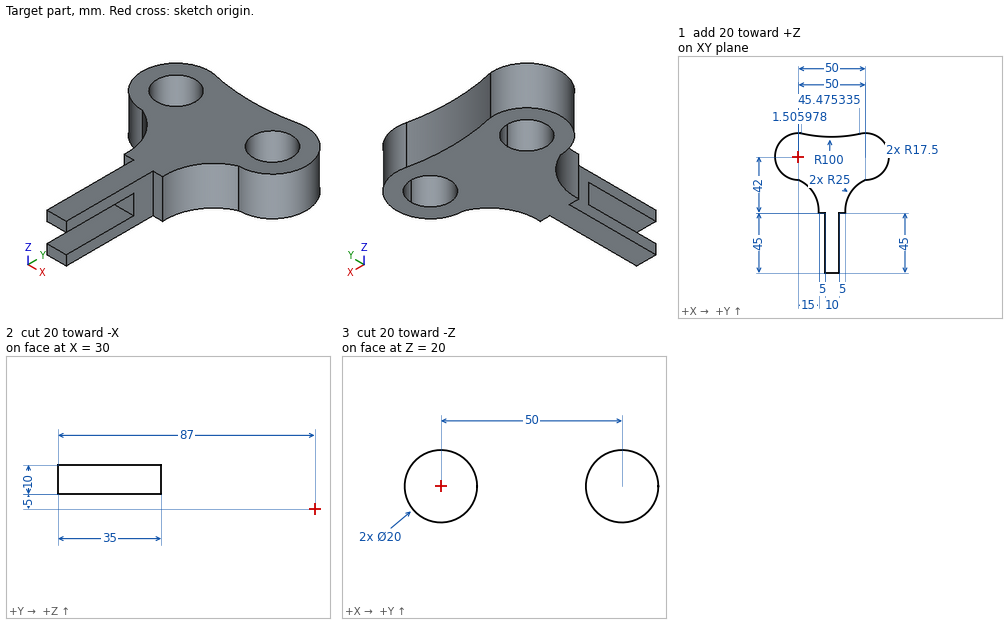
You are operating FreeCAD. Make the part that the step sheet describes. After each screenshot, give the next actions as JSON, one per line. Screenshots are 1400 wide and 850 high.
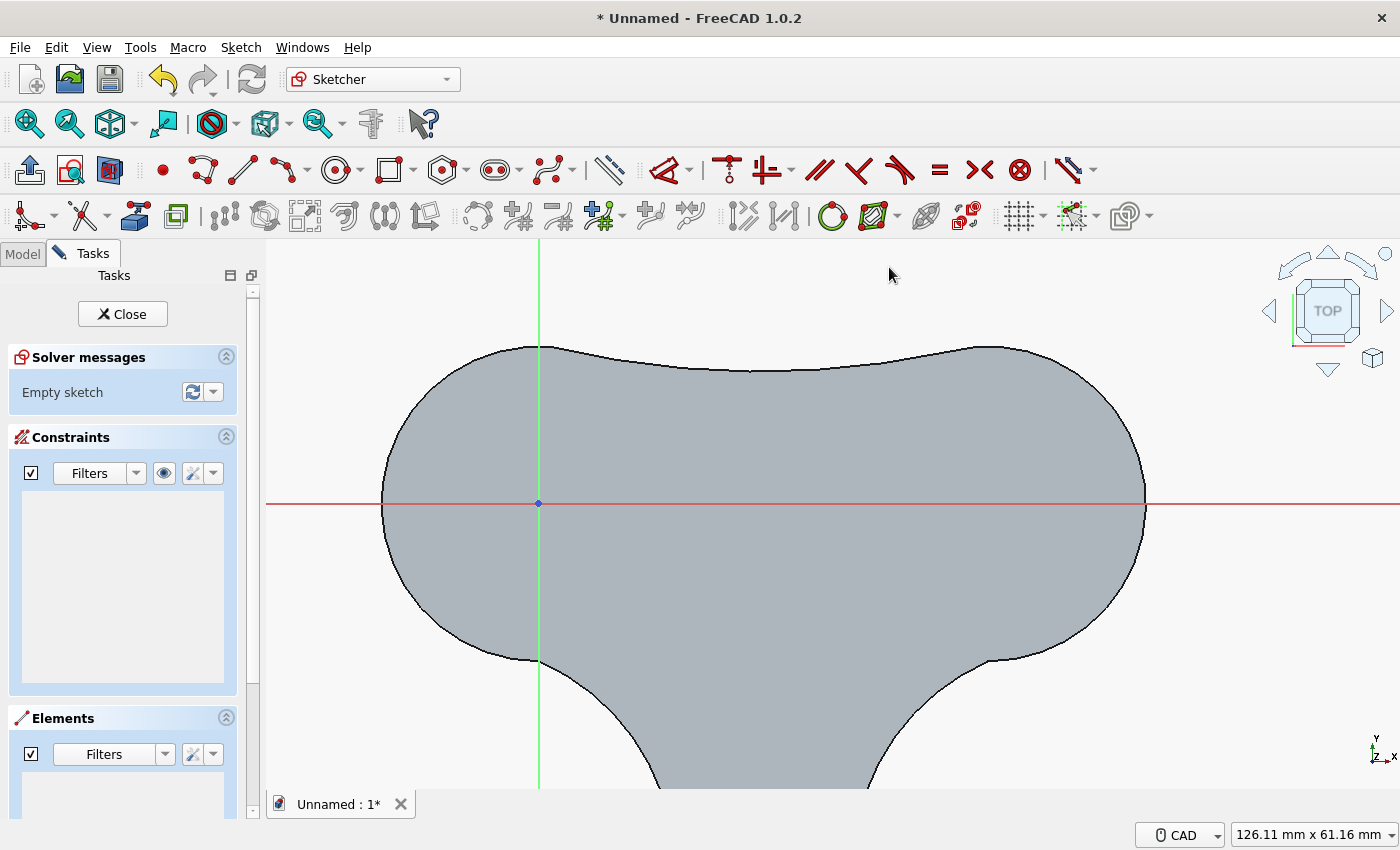
{"action": "left_click", "coordinate": [336, 170]}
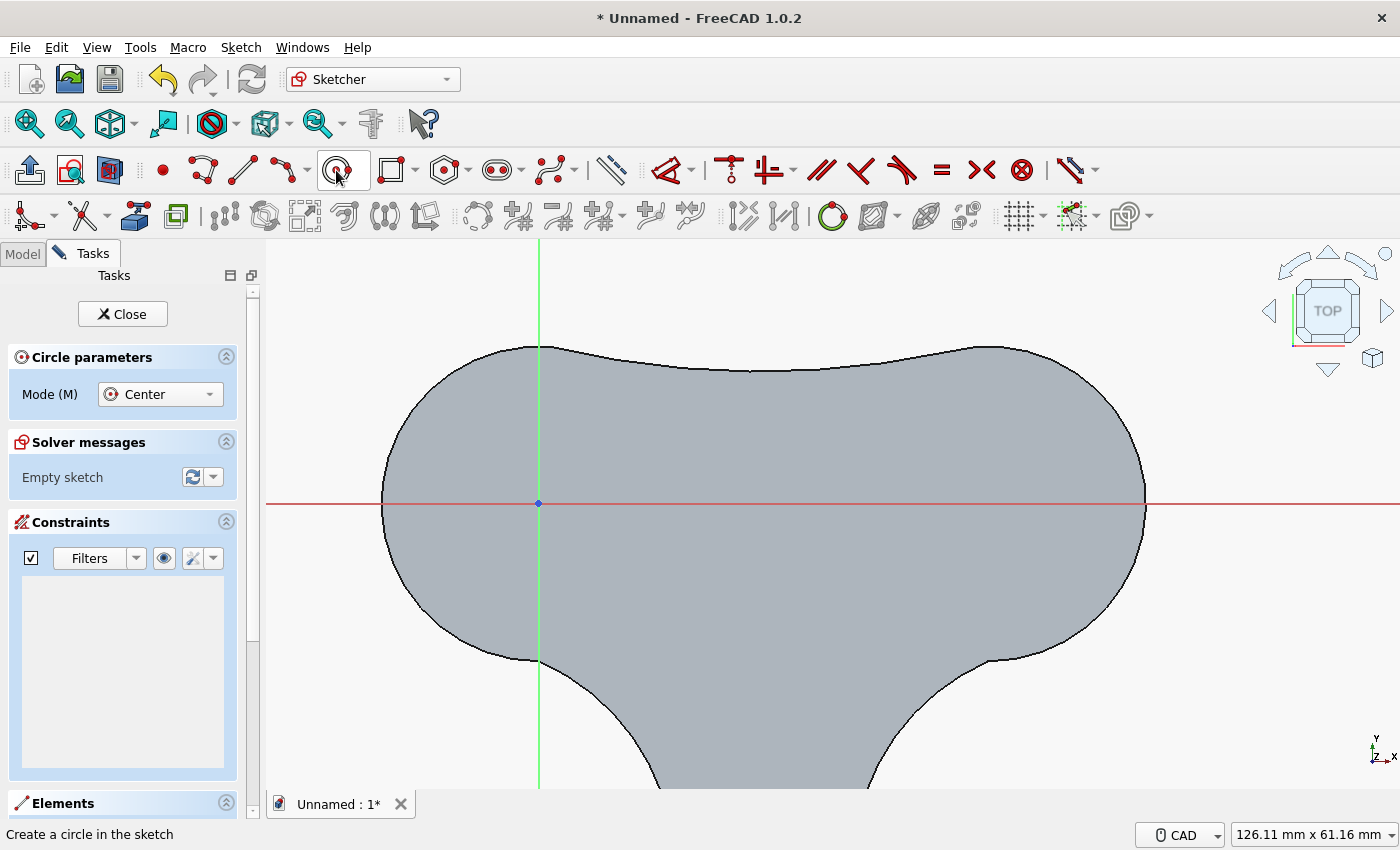
{"action": "left_click", "coordinate": [539, 504]}
{"action": "left_click", "coordinate": [602, 440]}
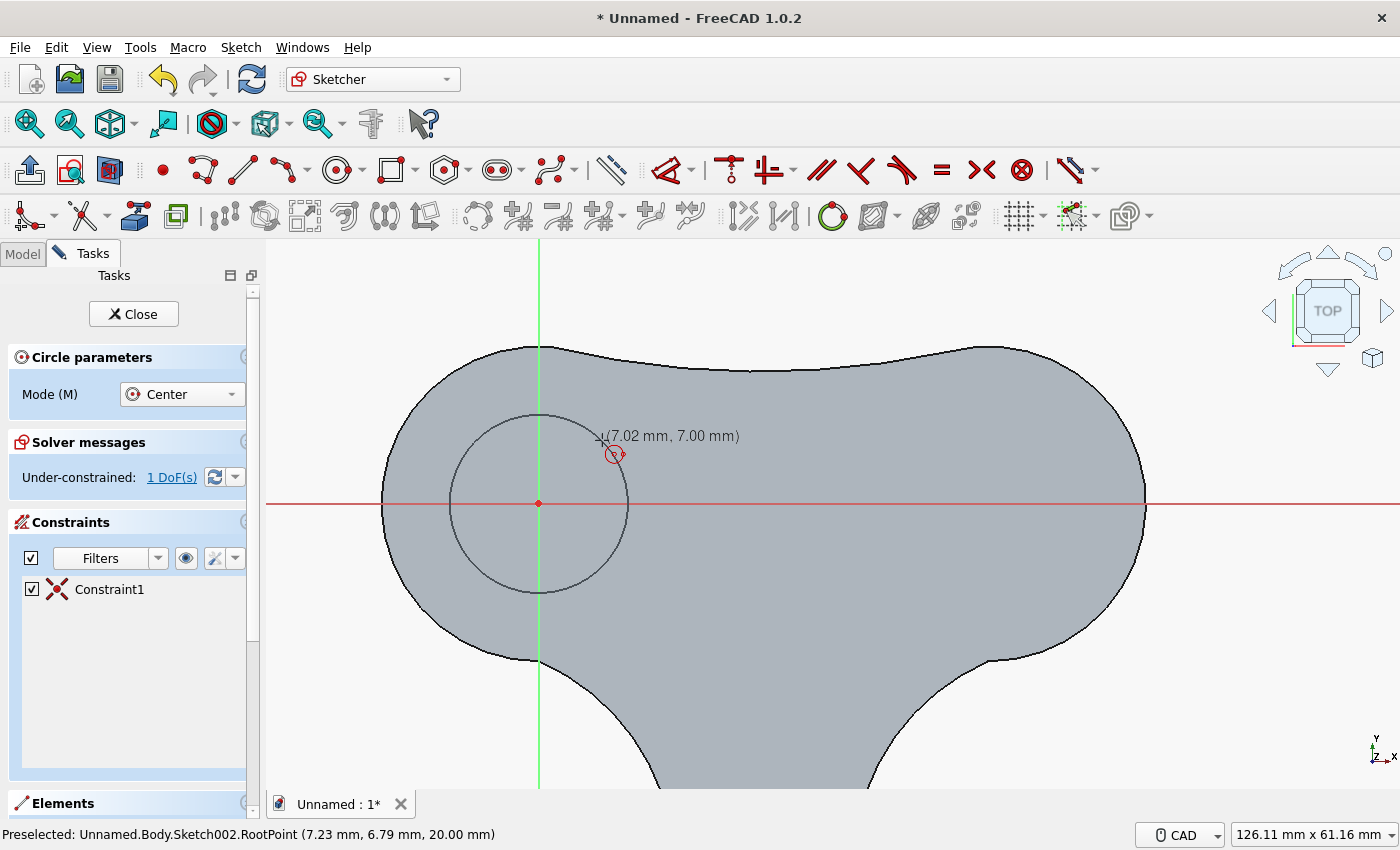
{"action": "left_click", "coordinate": [988, 504]}
{"action": "left_click", "coordinate": [1052, 440]}
{"action": "key", "text": "Escape"}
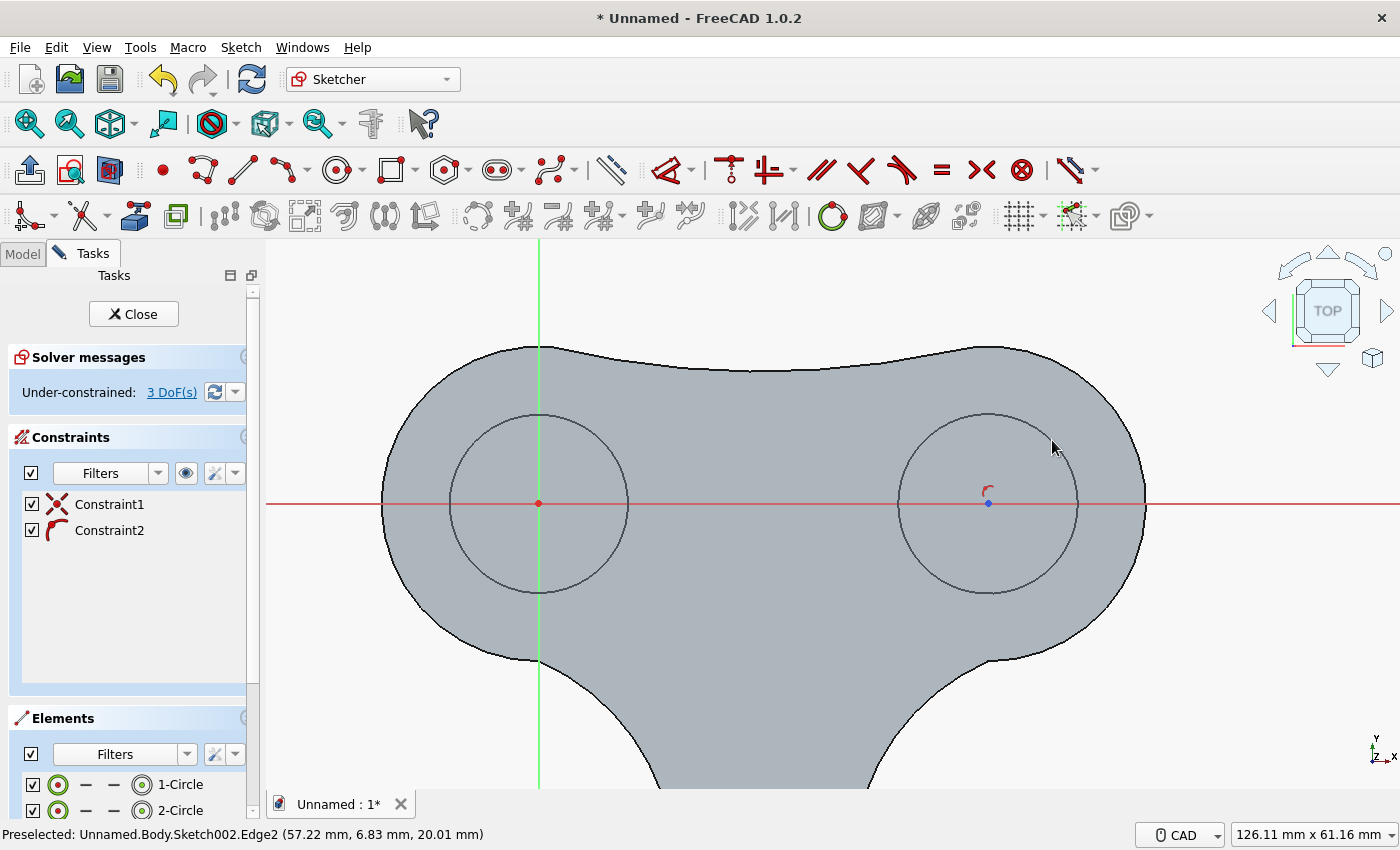
{"action": "left_click", "coordinate": [602, 441]}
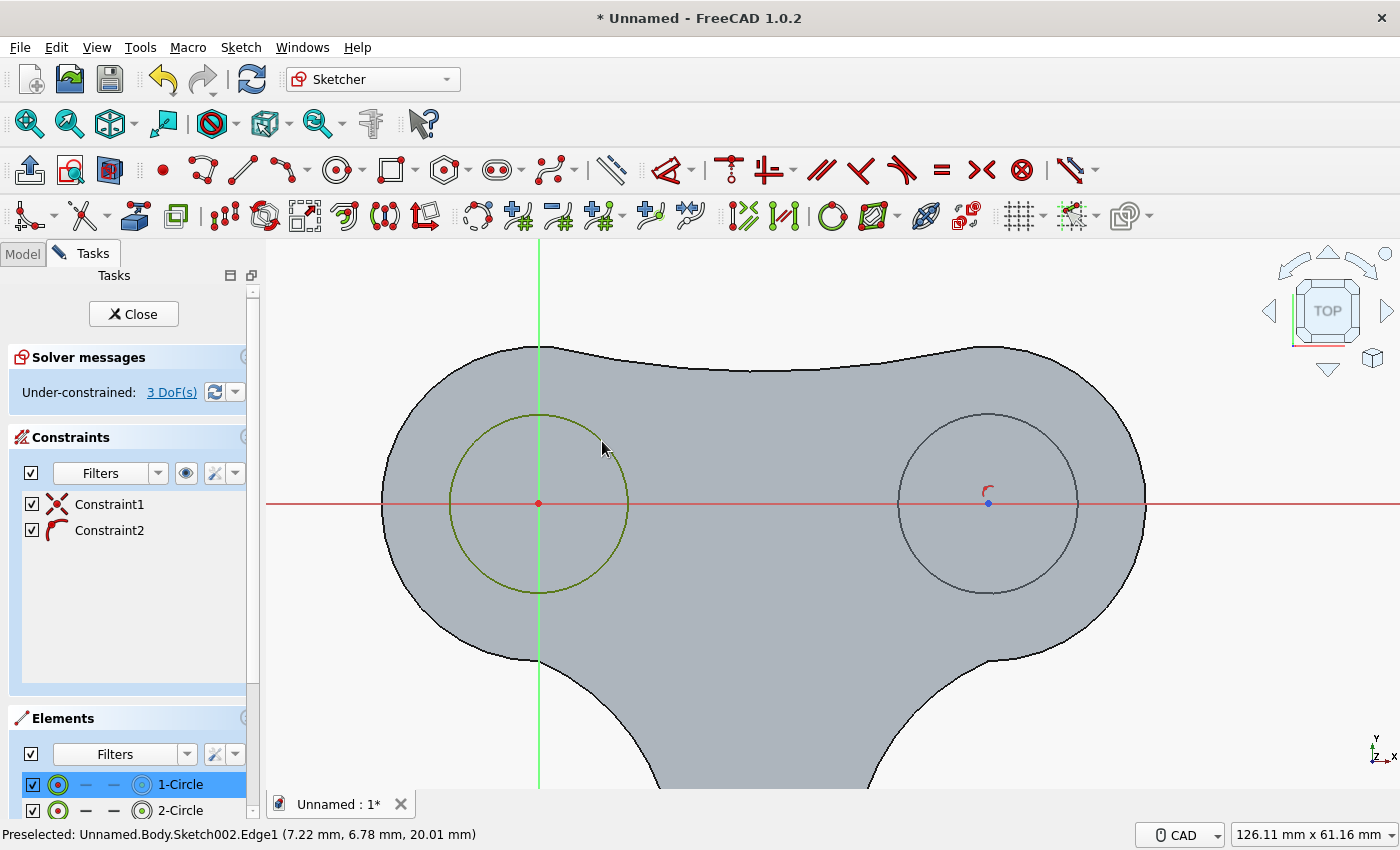
{"action": "left_click", "coordinate": [1051, 440]}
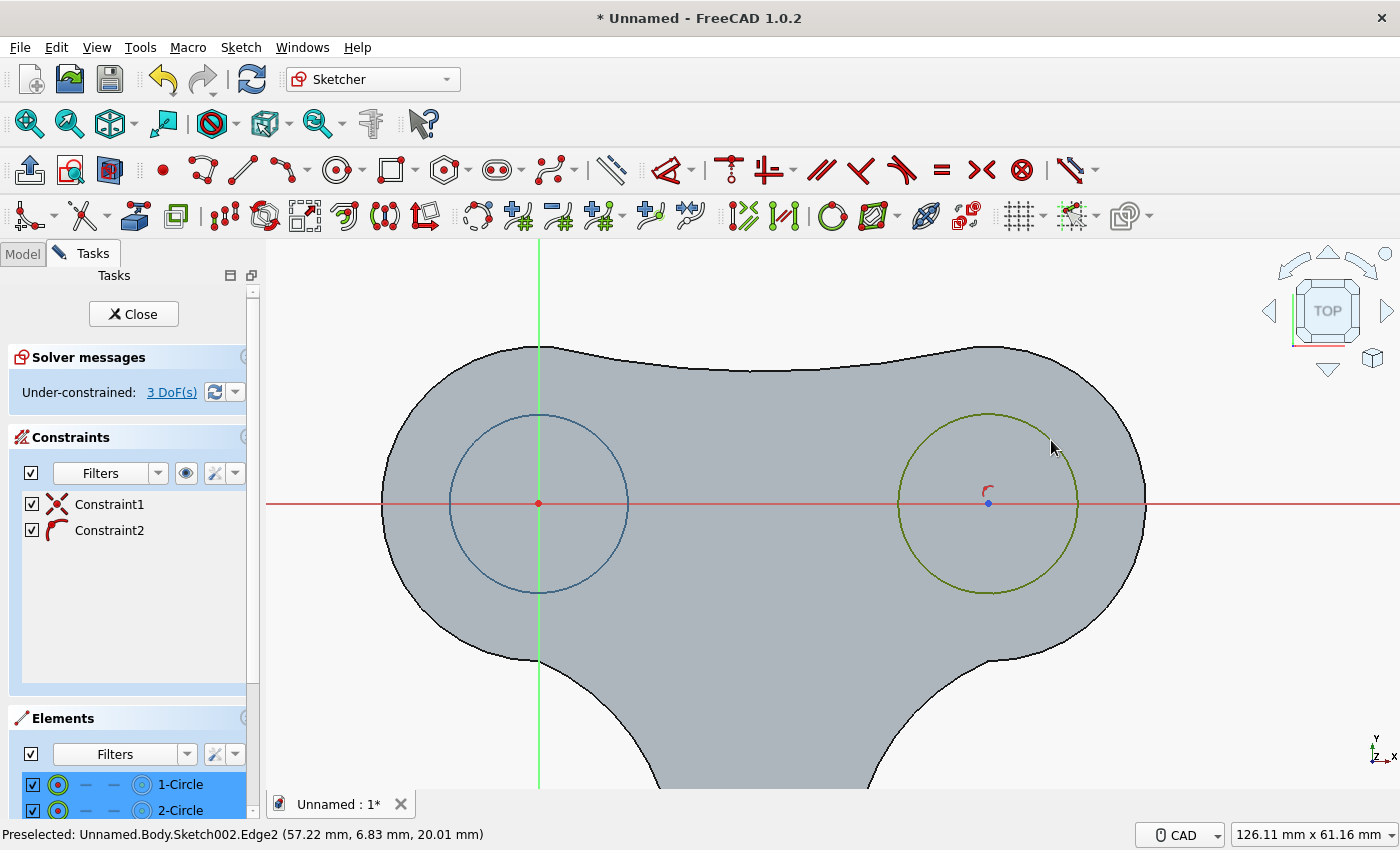
{"action": "left_click", "coordinate": [942, 170]}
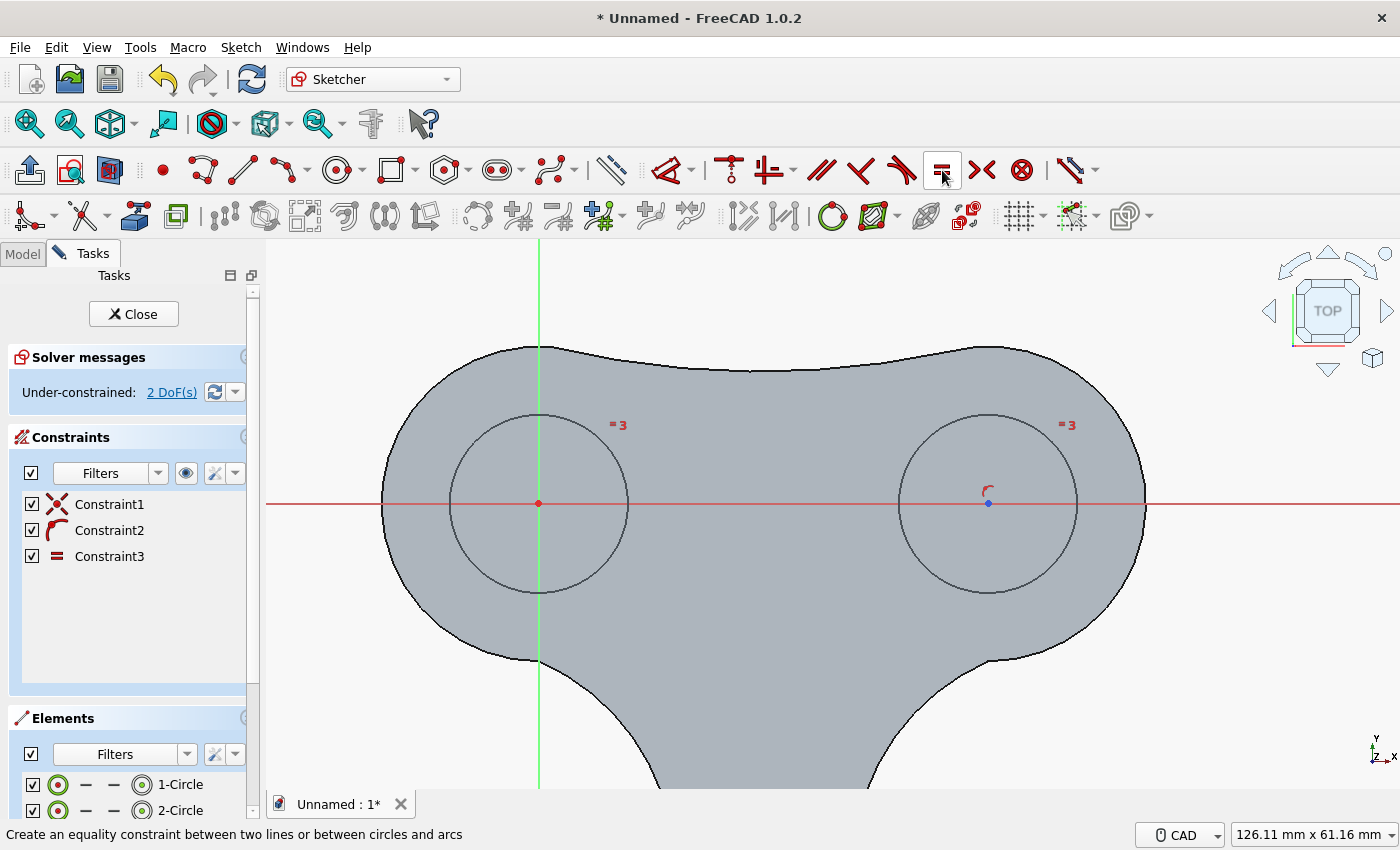
{"action": "left_click", "coordinate": [666, 170]}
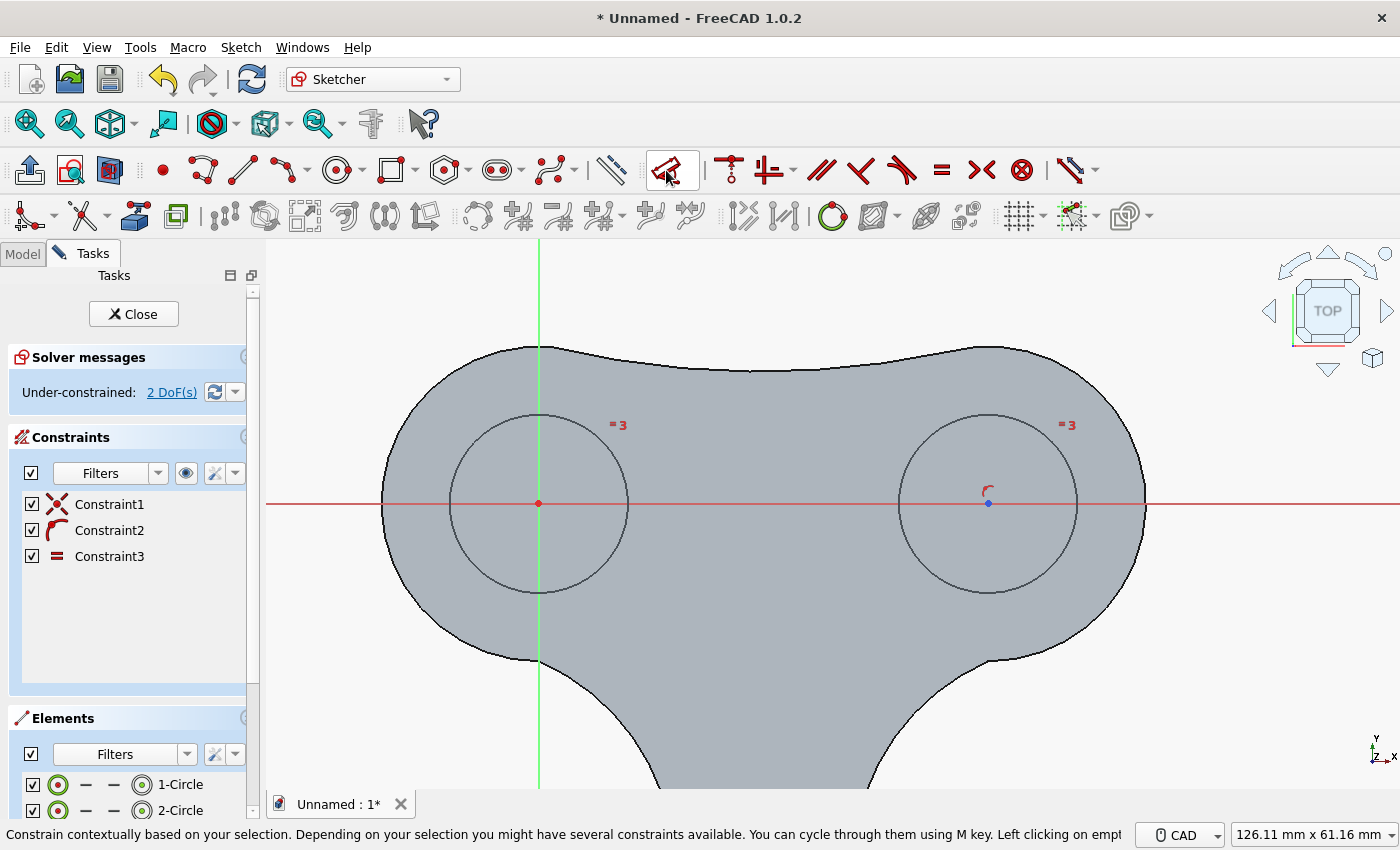
{"action": "left_click", "coordinate": [602, 441]}
{"action": "left_click", "coordinate": [625, 418]}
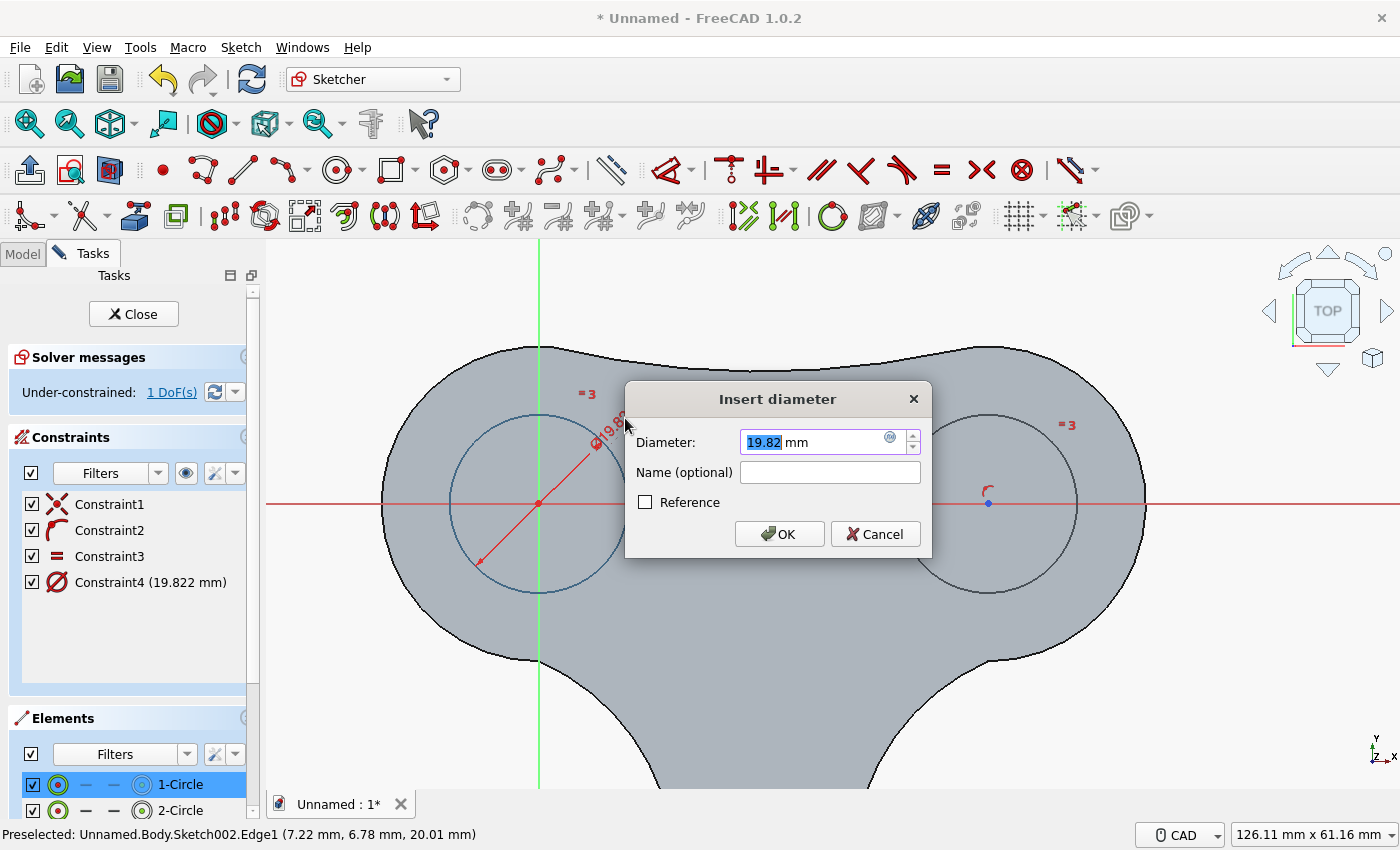
{"action": "type", "text": "20"}
{"action": "key", "text": "Return"}